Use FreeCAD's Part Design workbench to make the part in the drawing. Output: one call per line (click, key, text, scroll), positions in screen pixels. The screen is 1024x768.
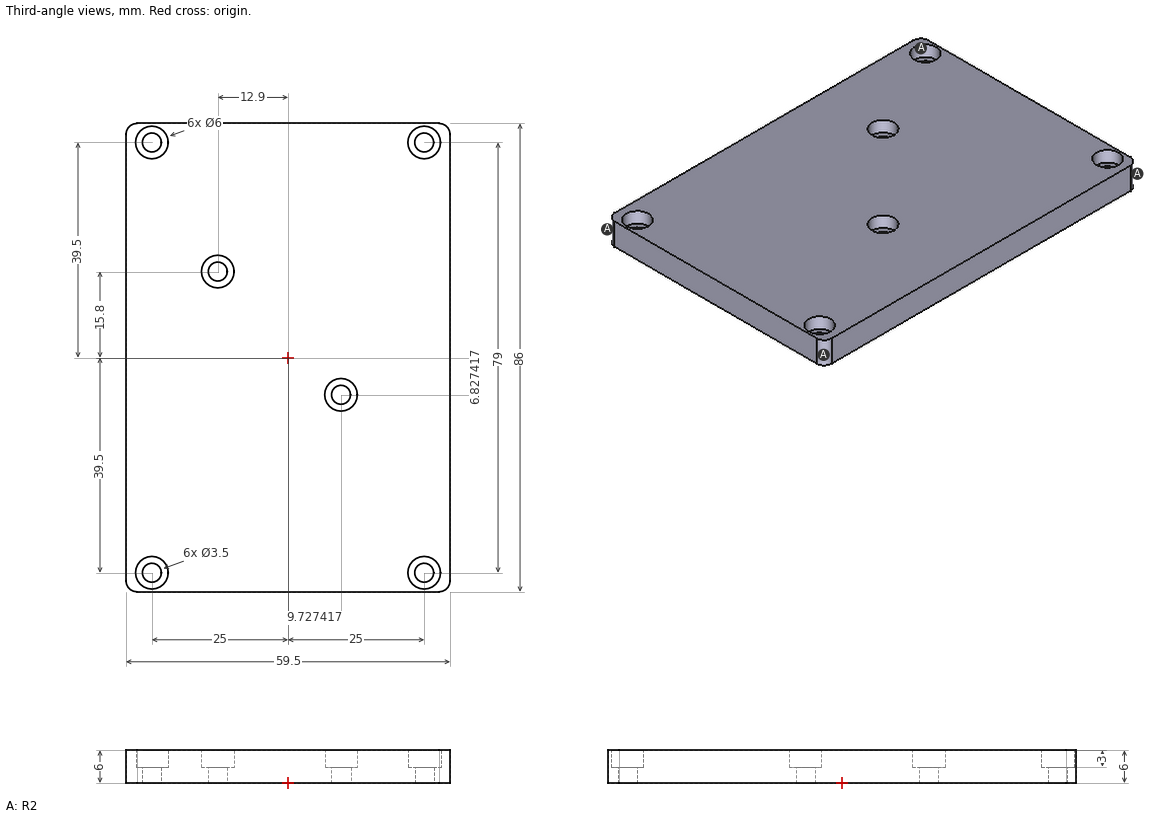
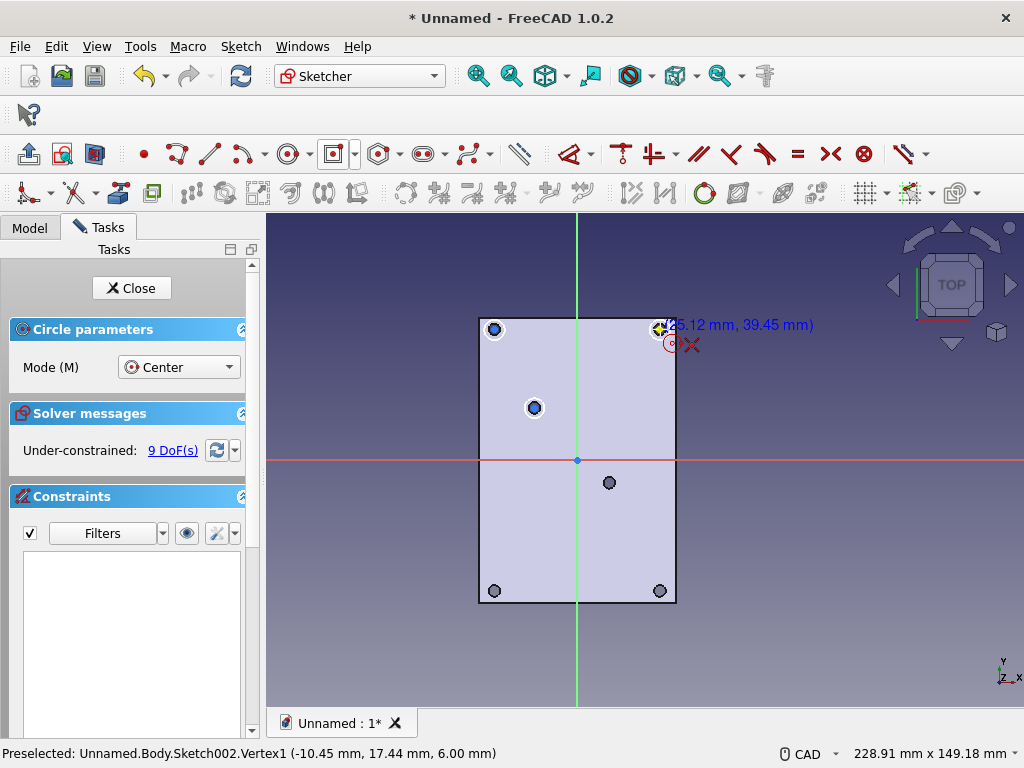
scroll(609, 483, up, 5)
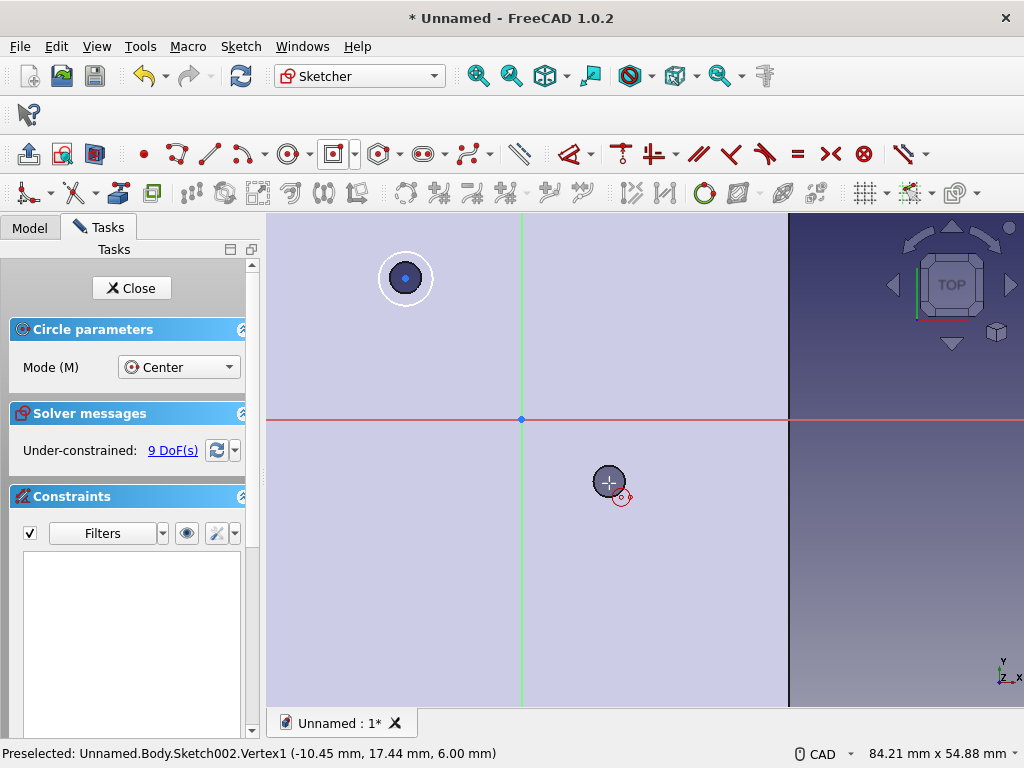
click(609, 481)
click(628, 462)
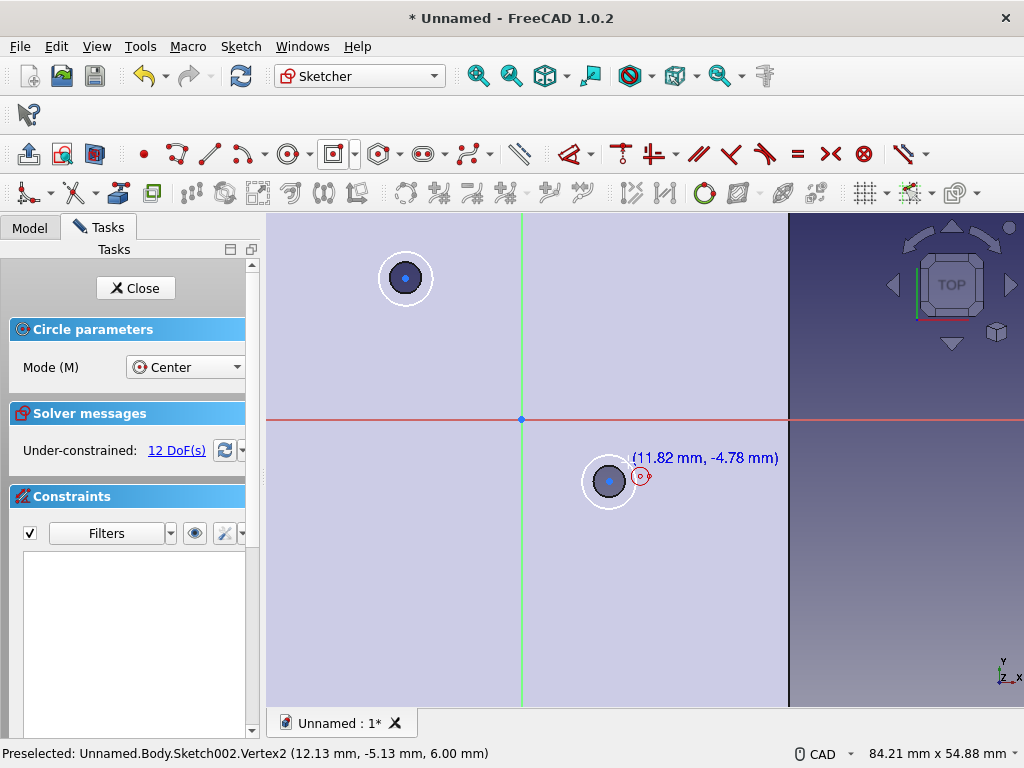
scroll(608, 483, down, 5)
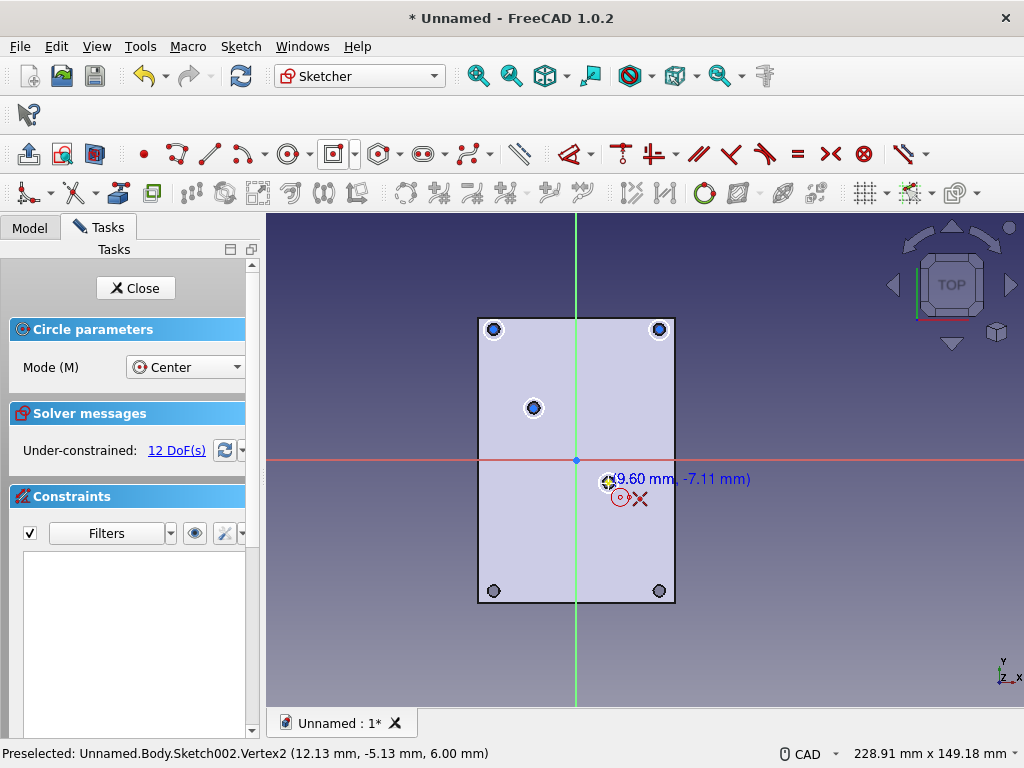
scroll(494, 591, up, 5)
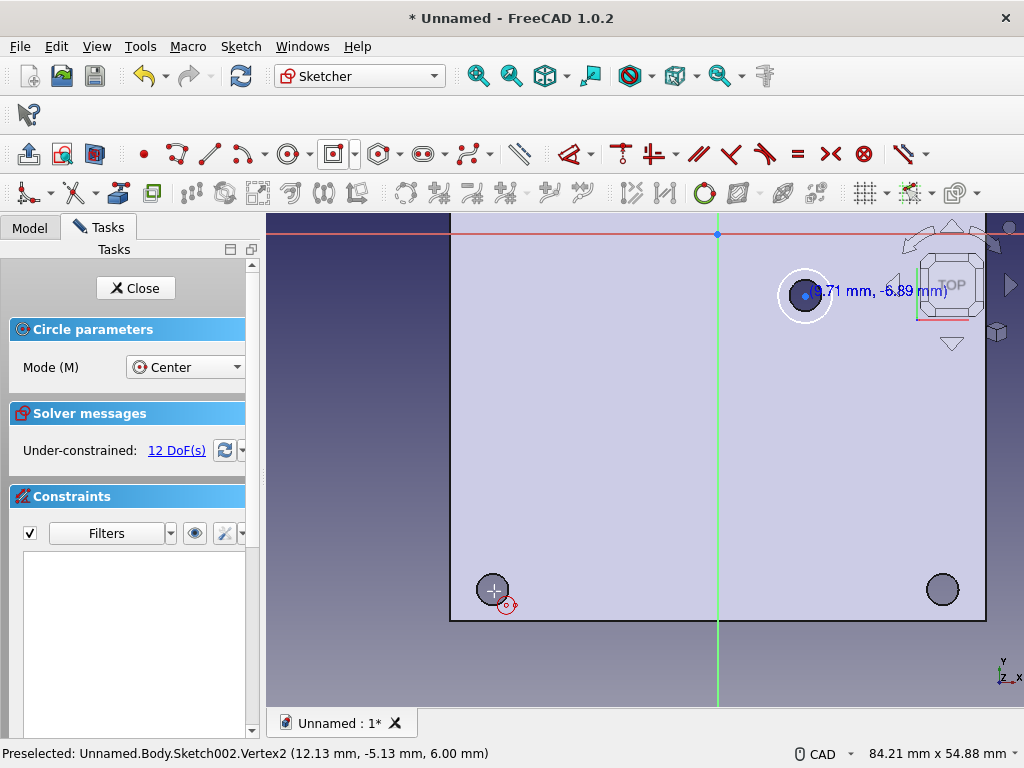
click(493, 590)
click(512, 570)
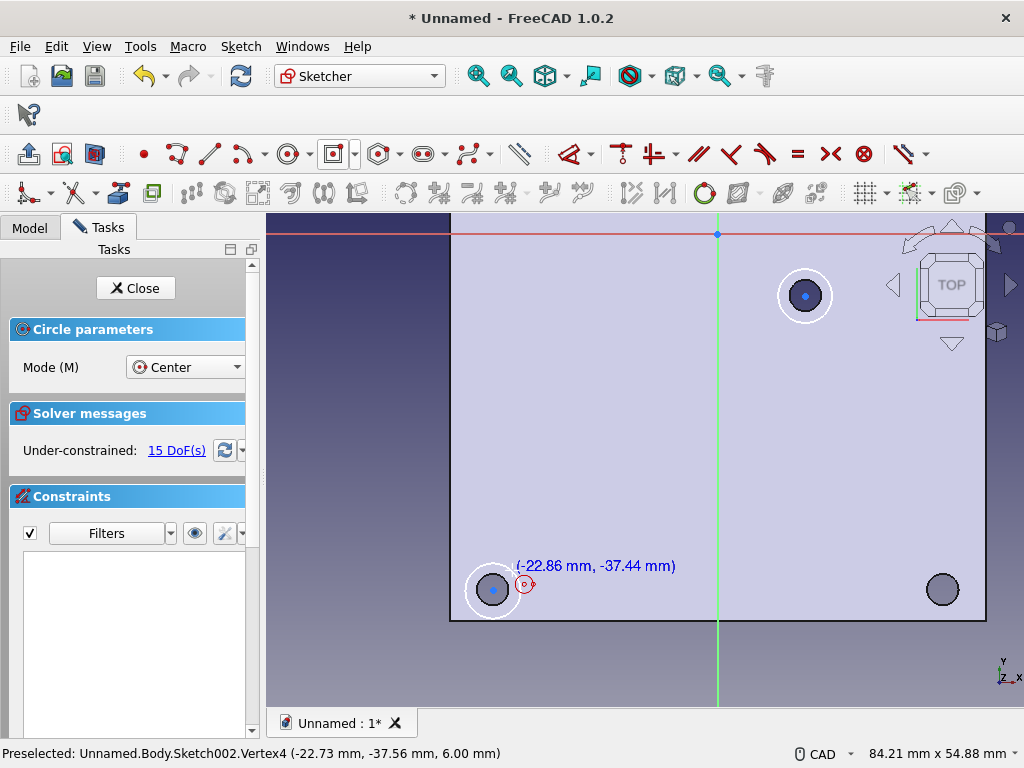
scroll(494, 592, down, 5)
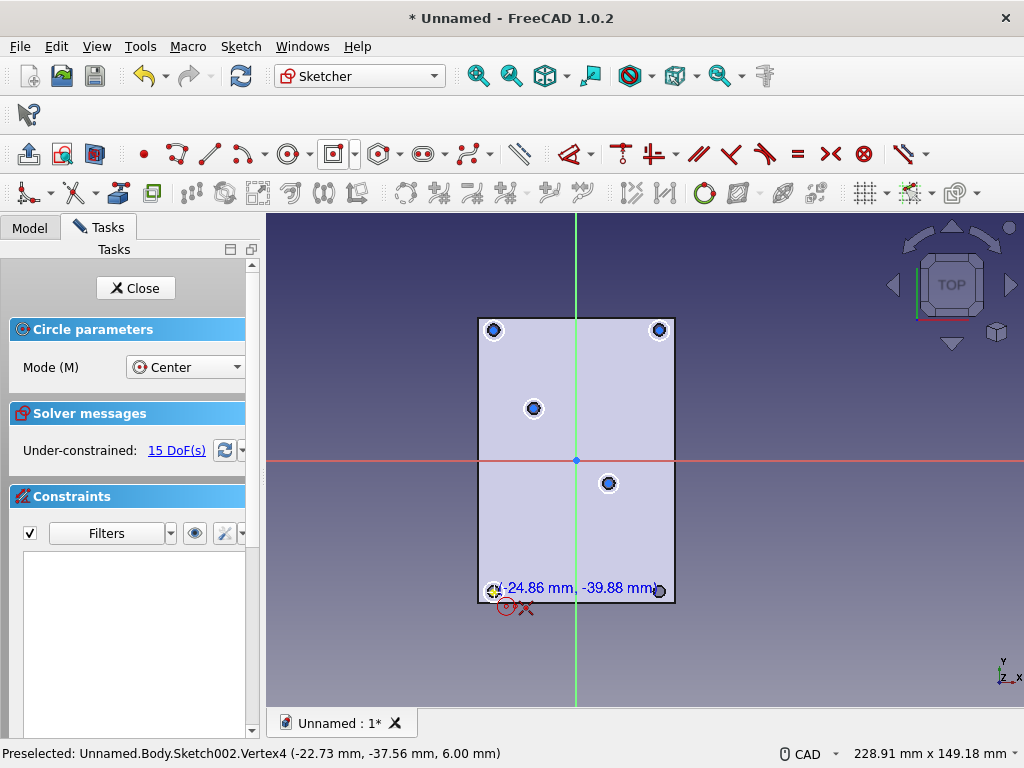
scroll(659, 592, up, 5)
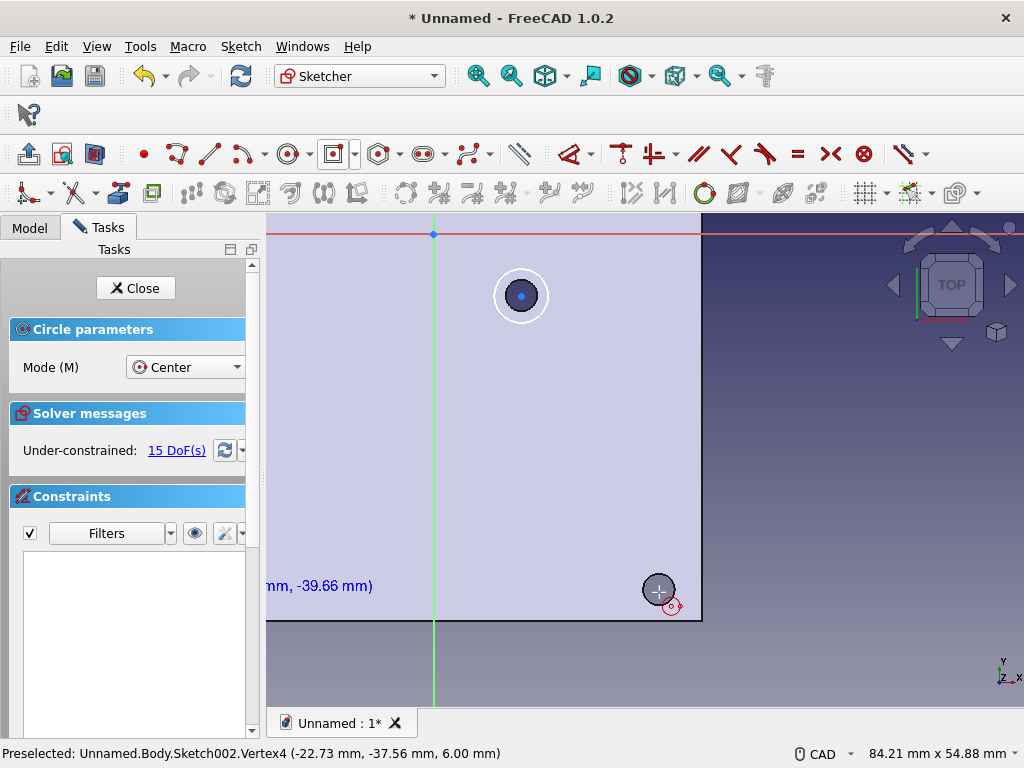
click(659, 590)
click(678, 570)
key(Escape)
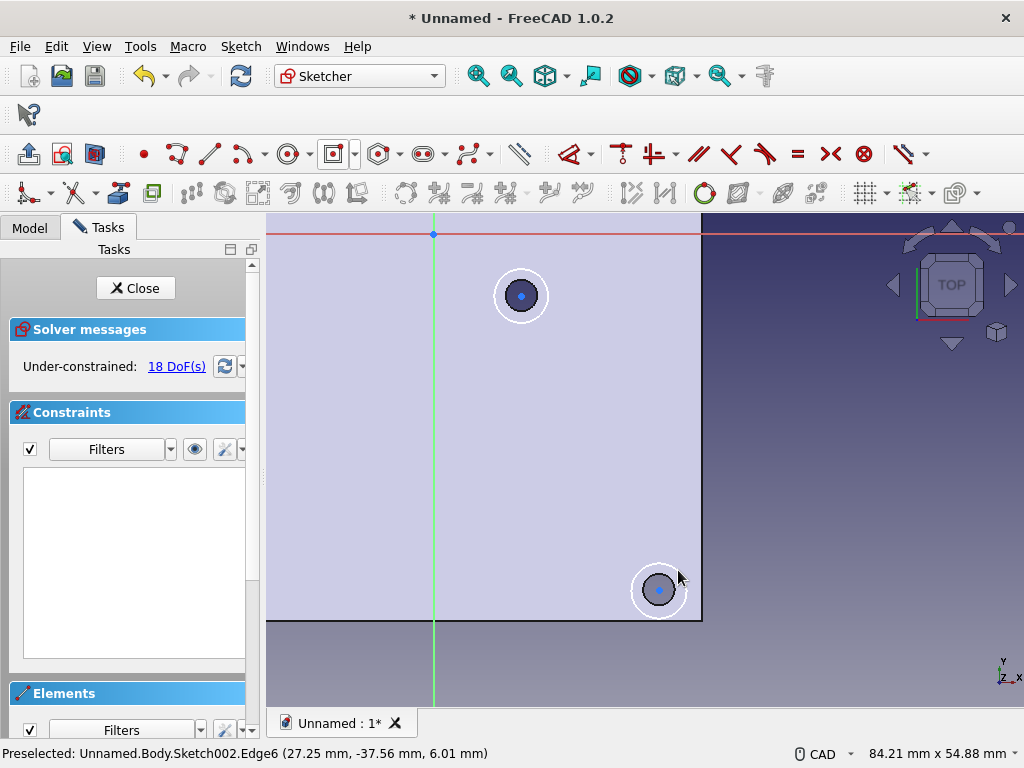
scroll(660, 592, down, 5)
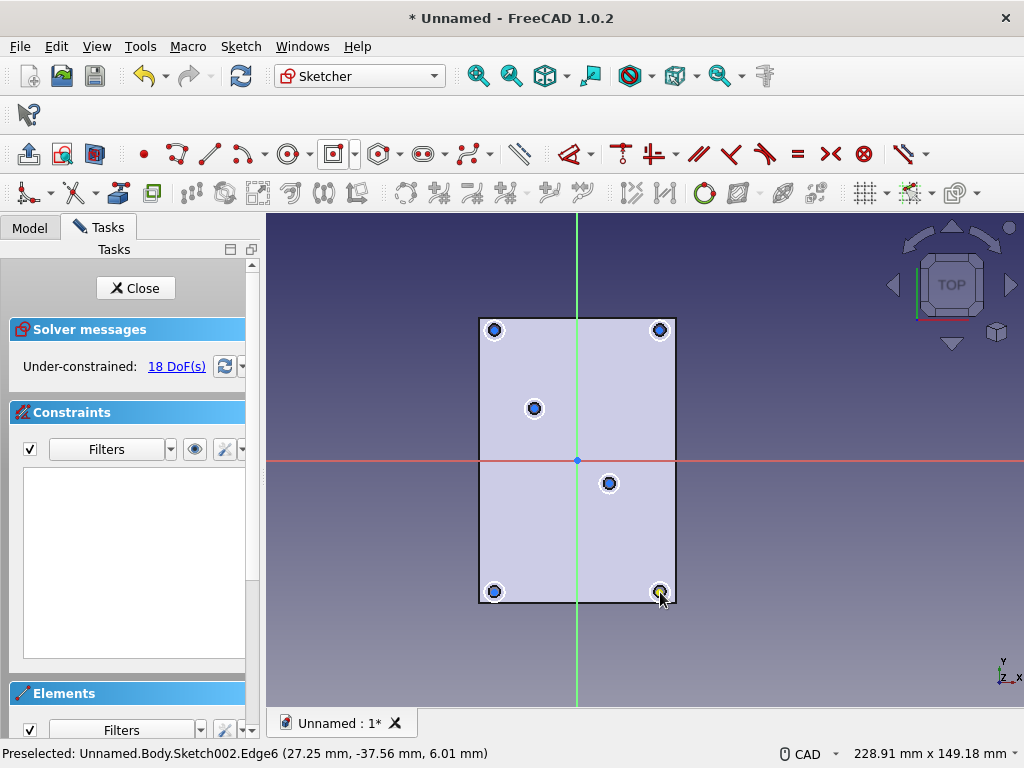
scroll(502, 323, up, 2)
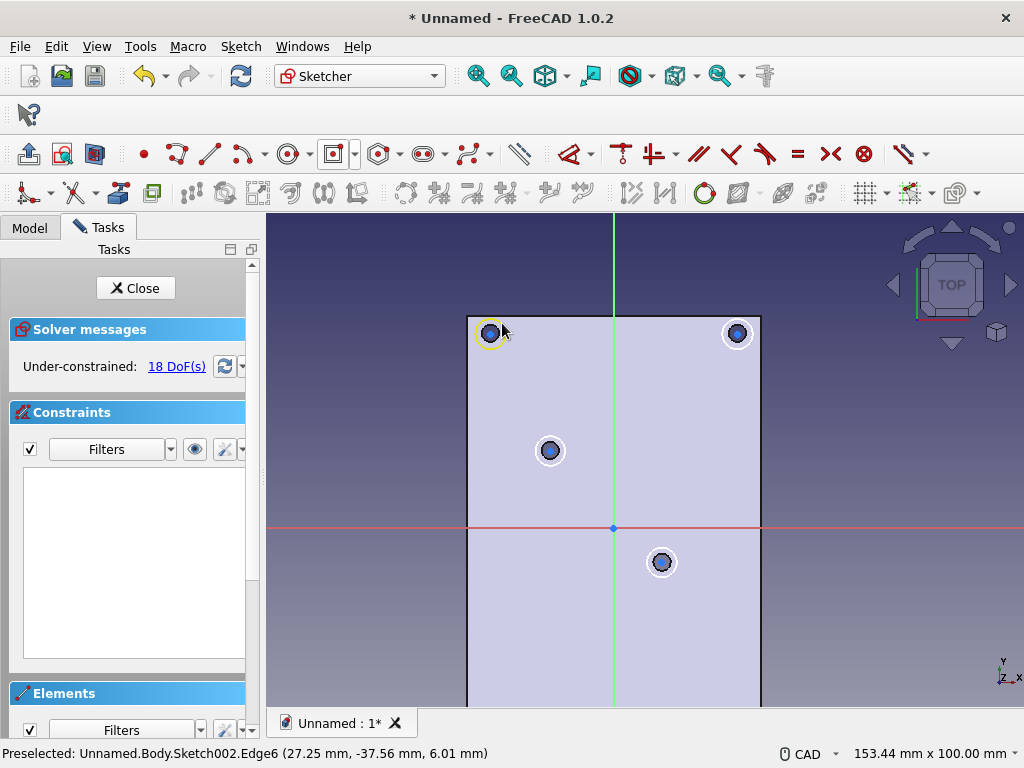
click(501, 323)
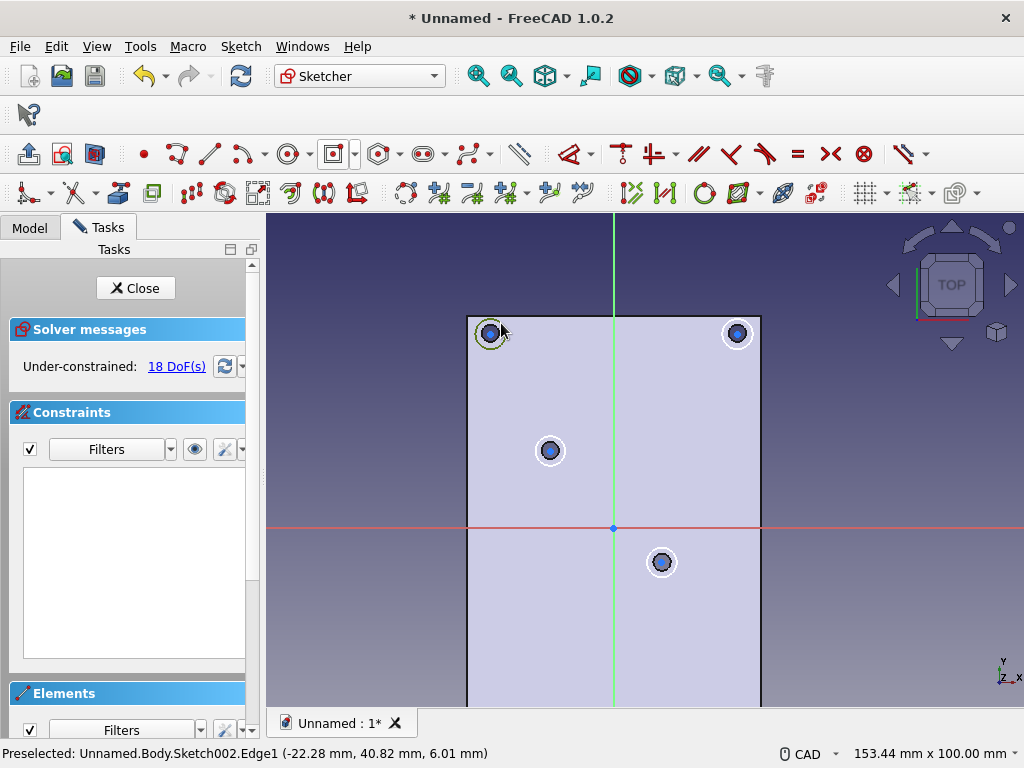
click(748, 323)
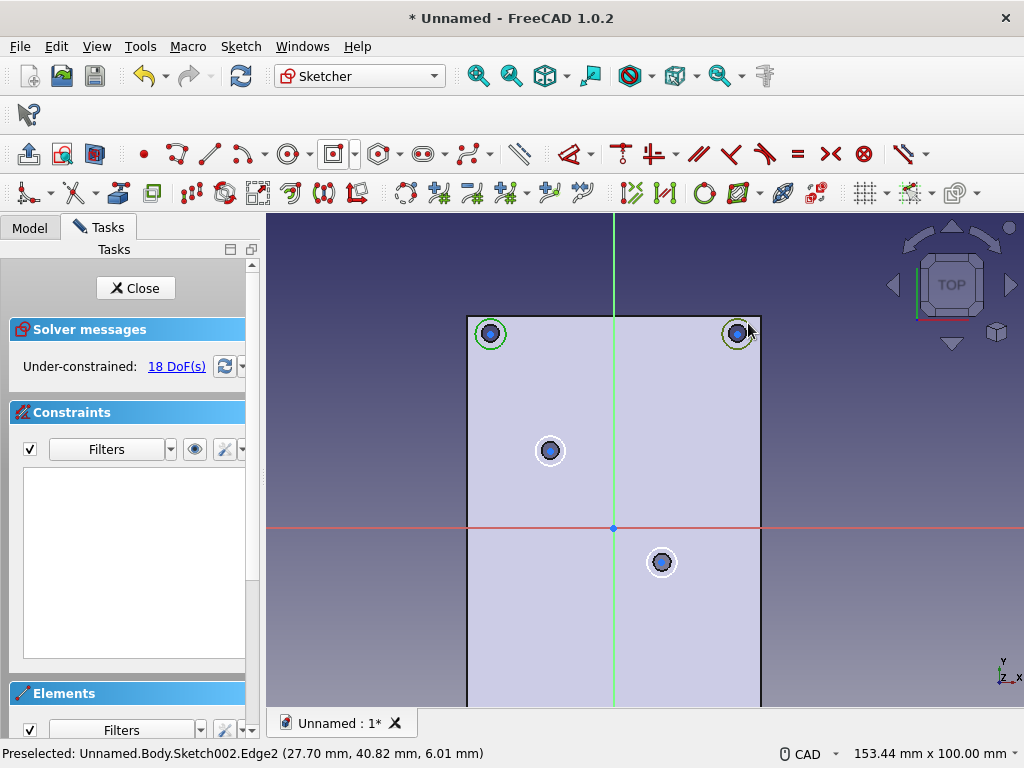
click(561, 441)